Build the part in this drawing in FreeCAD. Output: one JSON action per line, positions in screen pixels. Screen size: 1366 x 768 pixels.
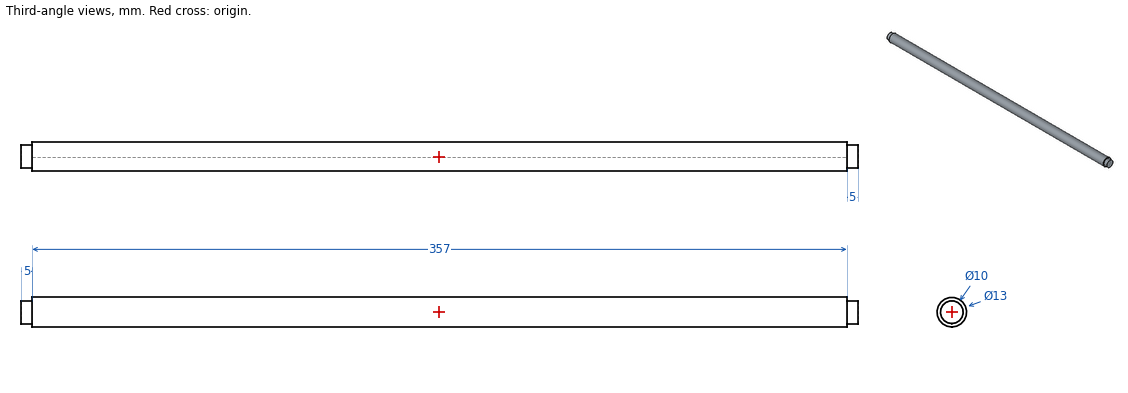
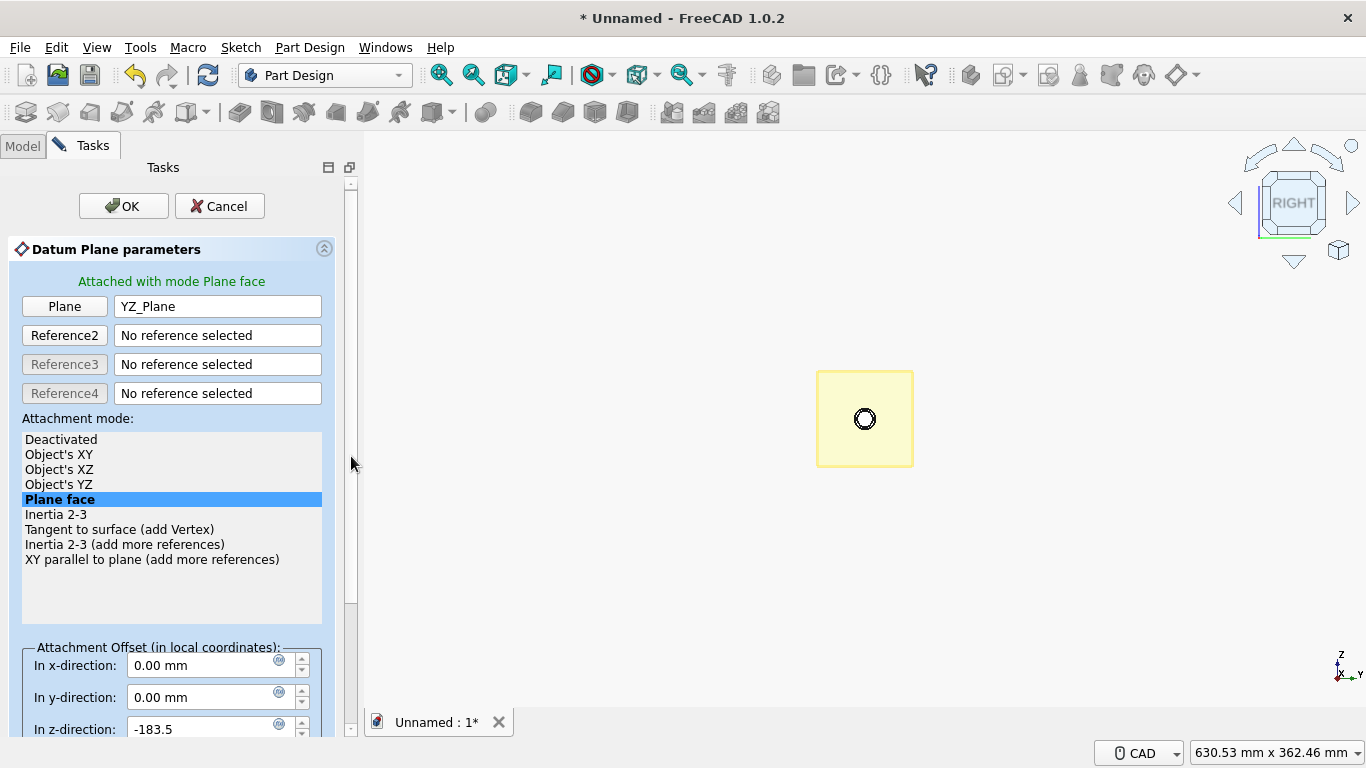
{"action": "left_click", "coordinate": [124, 206]}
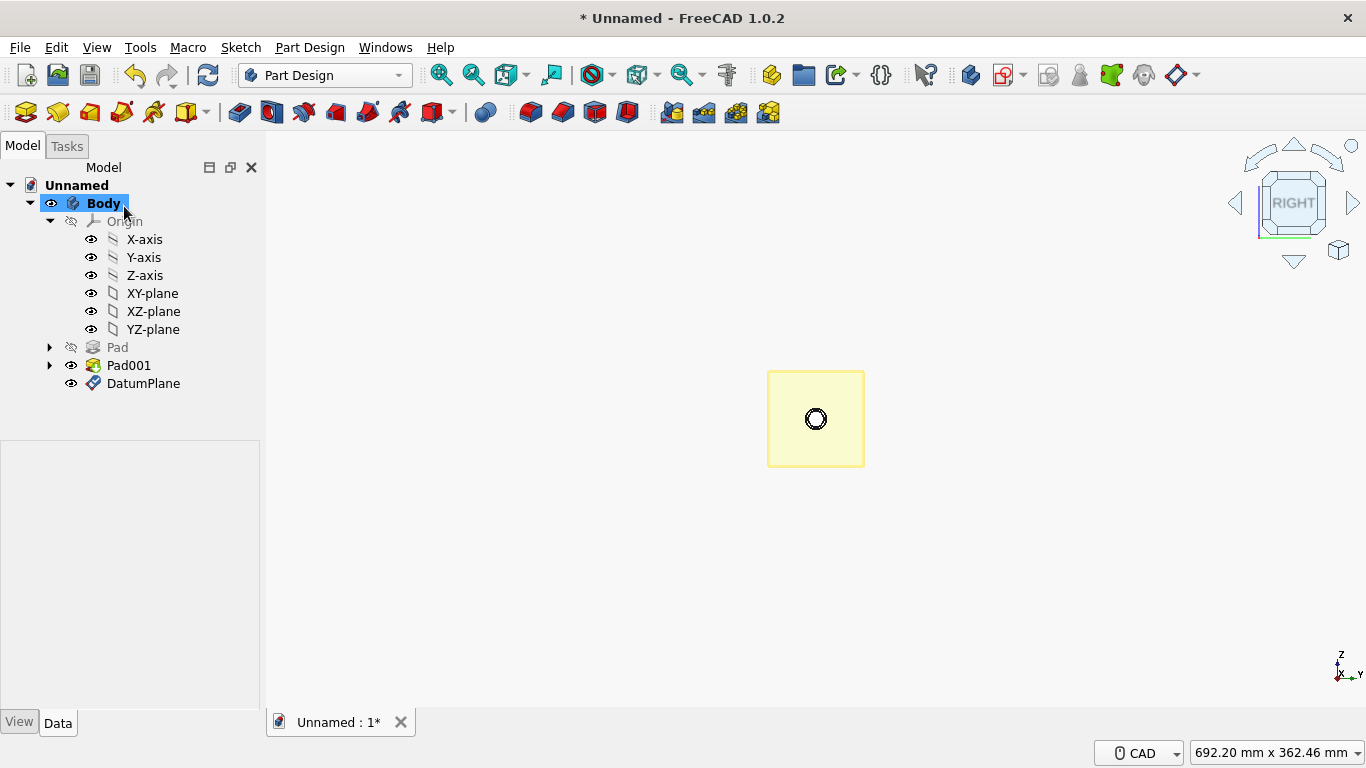
{"action": "left_click", "coordinate": [116, 383]}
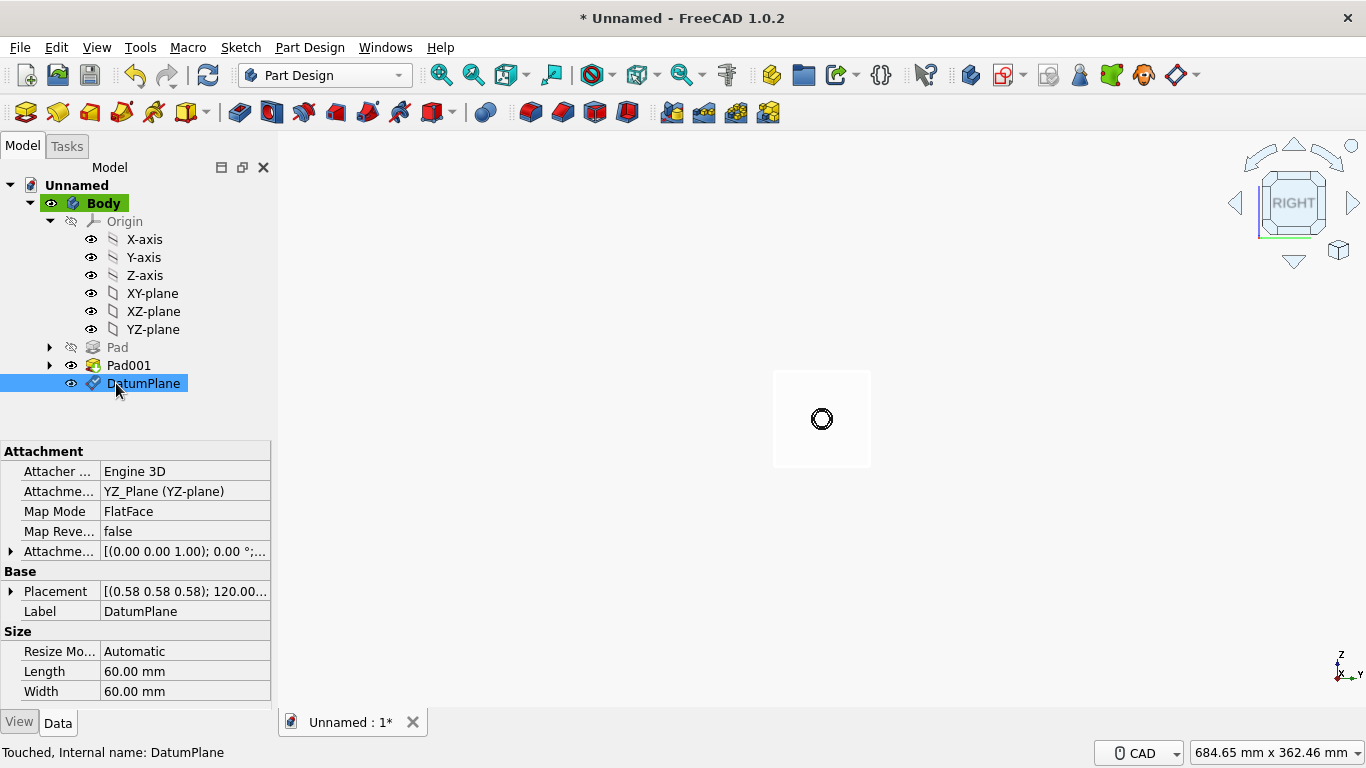
{"action": "left_click", "coordinate": [1004, 76]}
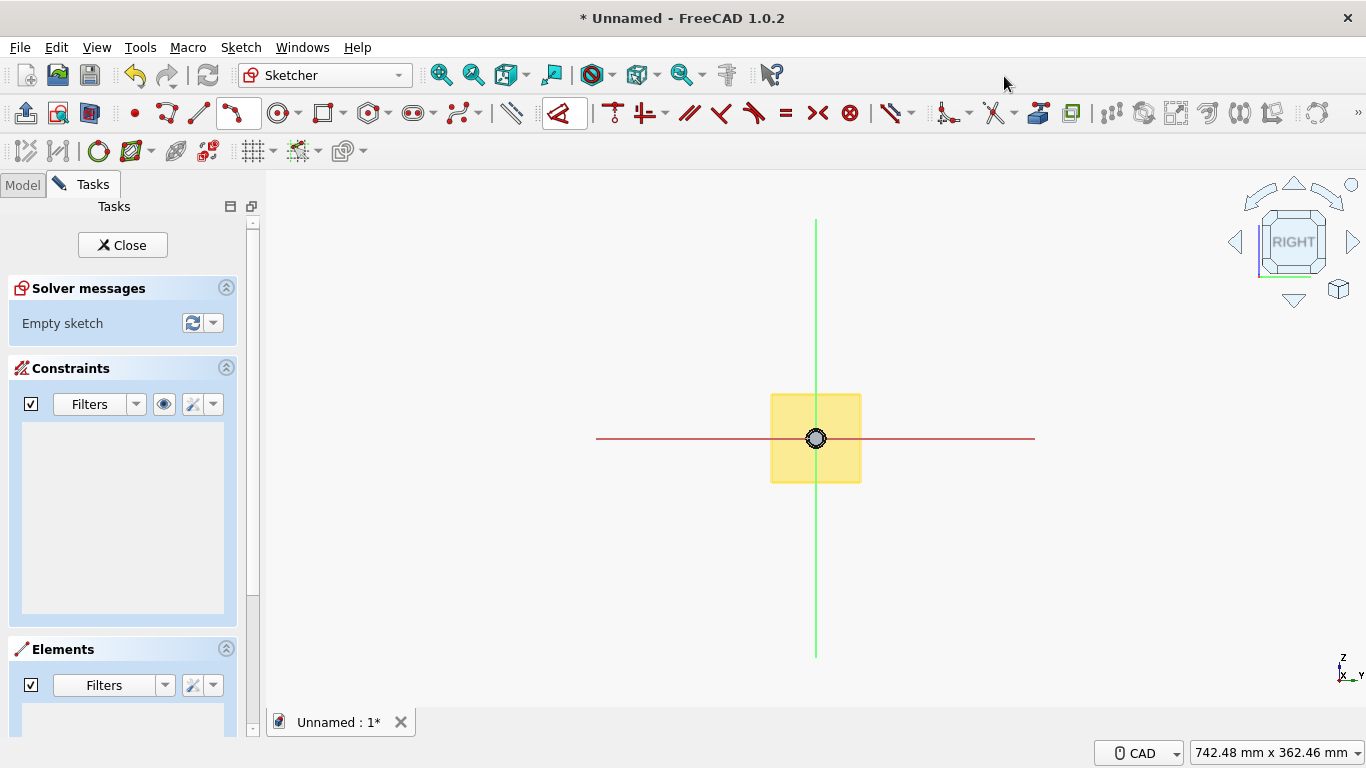
{"action": "left_click", "coordinate": [90, 114]}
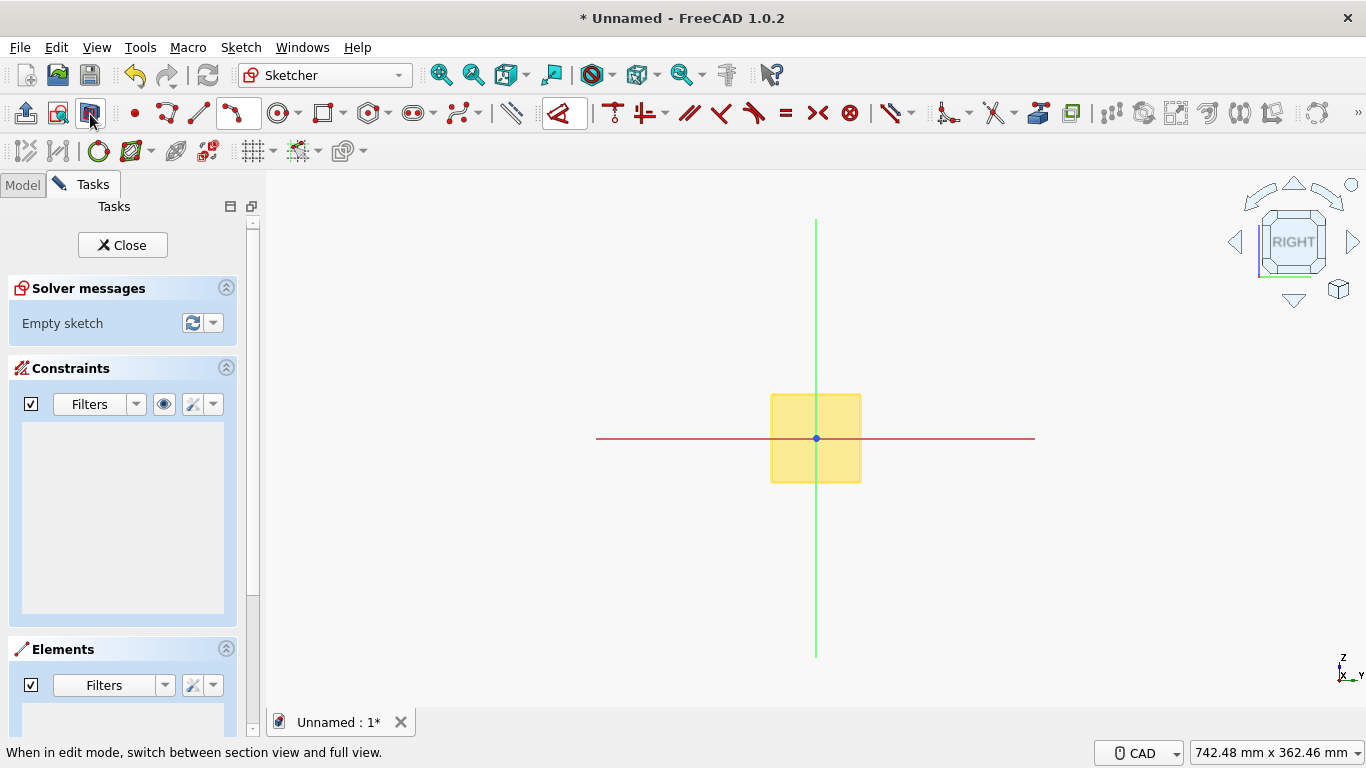
{"action": "scroll", "coordinate": [820, 438], "scroll_direction": "up", "scroll_amount": 15}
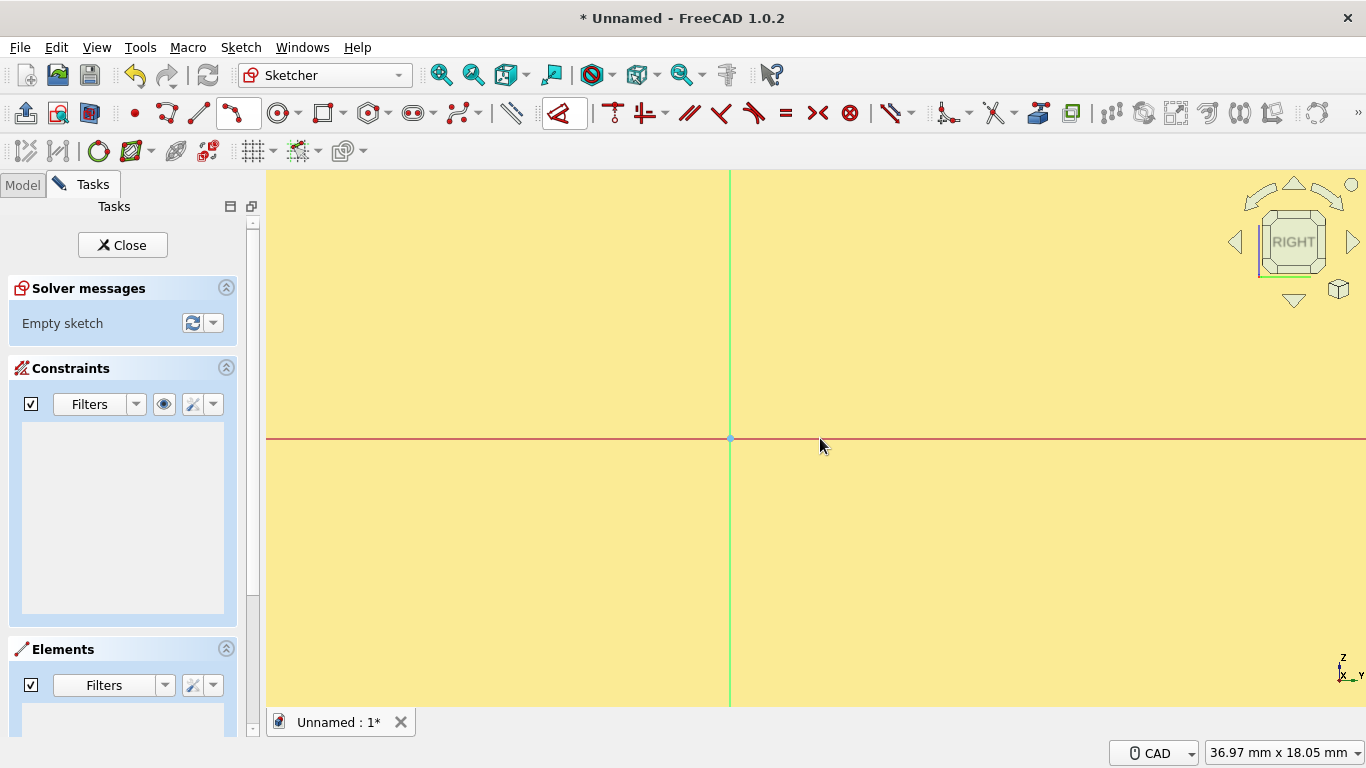
{"action": "left_click", "coordinate": [278, 114]}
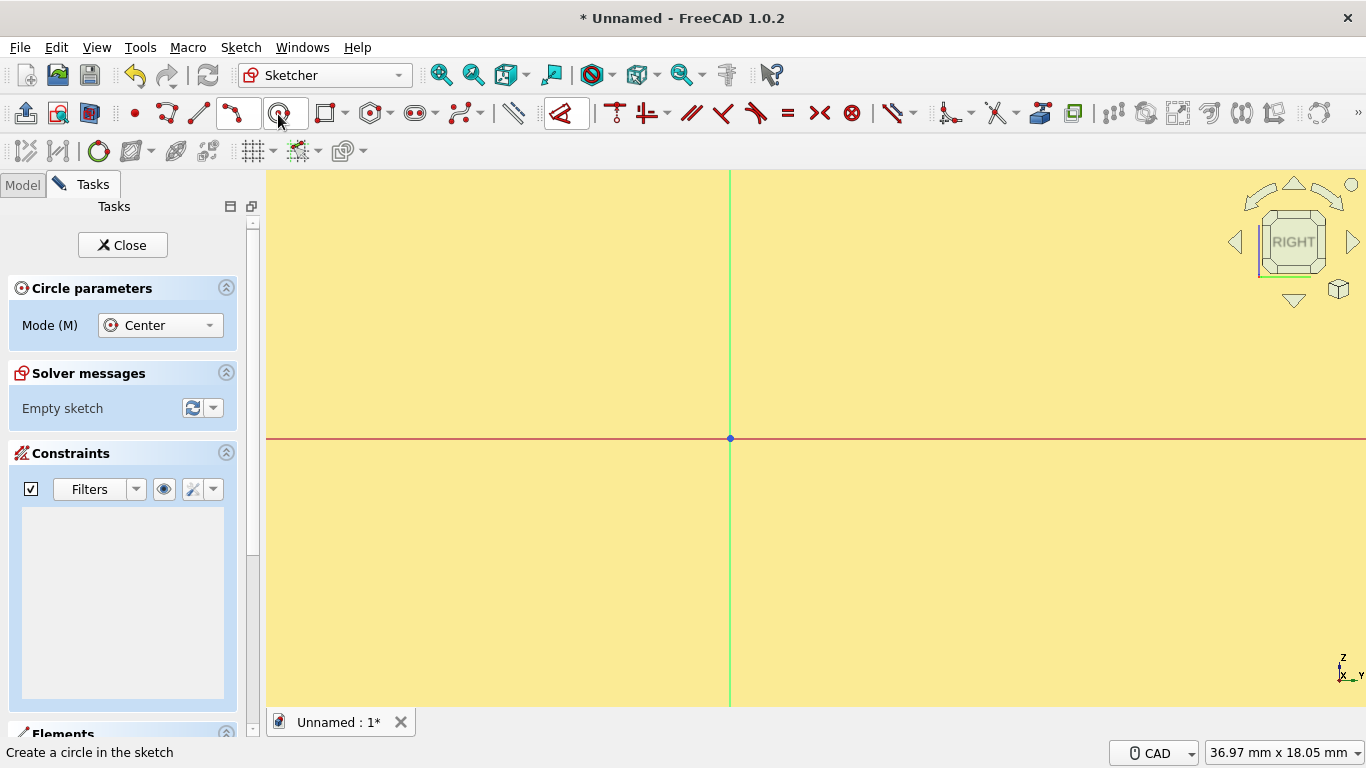
{"action": "left_click", "coordinate": [730, 438]}
{"action": "left_click", "coordinate": [835, 333]}
{"action": "key", "text": "Escape"}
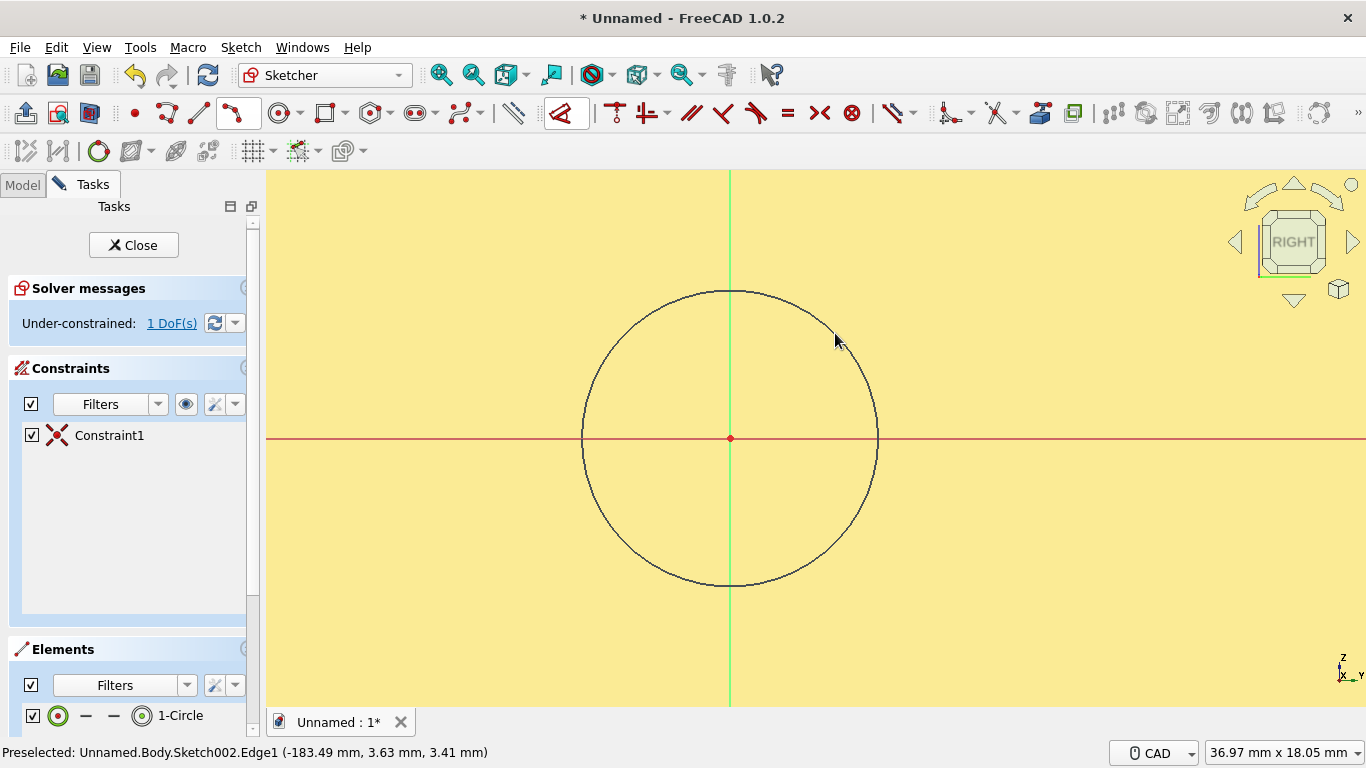
{"action": "left_click", "coordinate": [834, 333]}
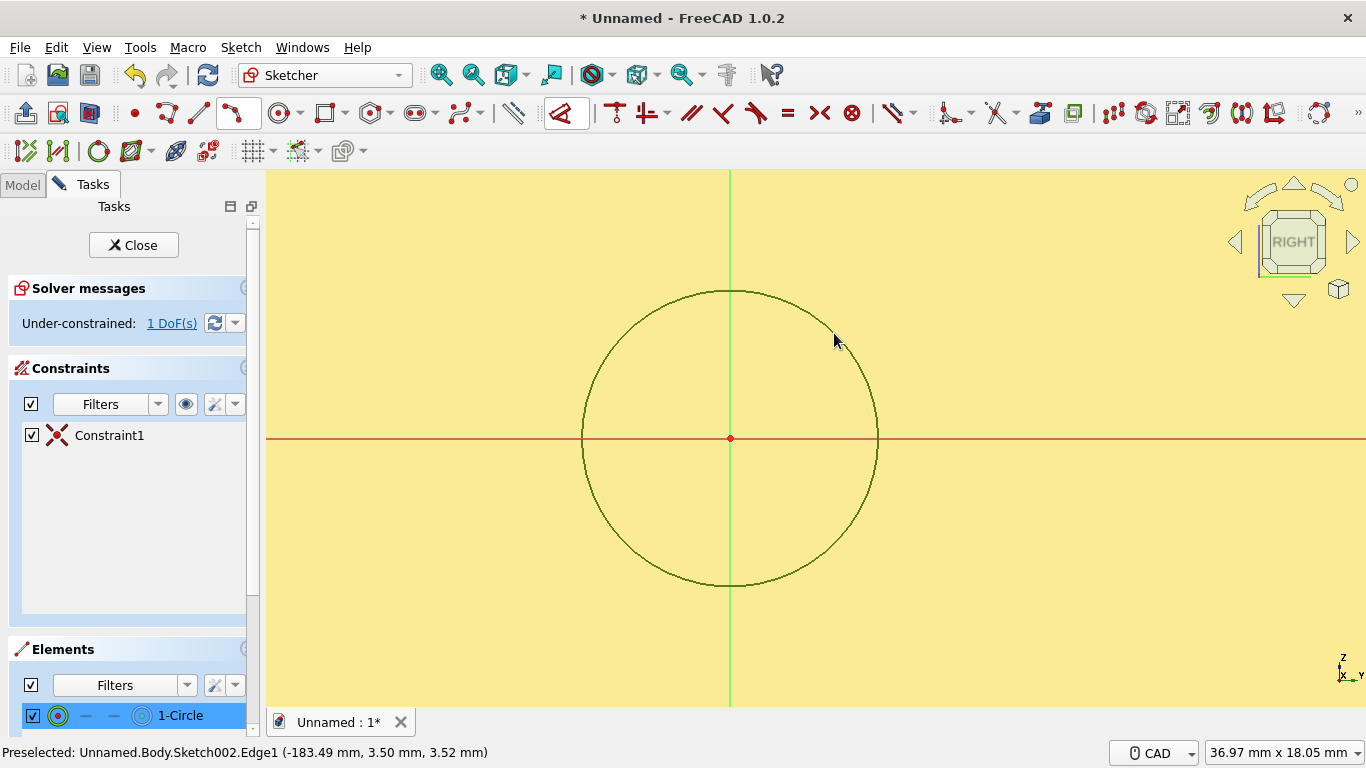
{"action": "left_click", "coordinate": [584, 114]}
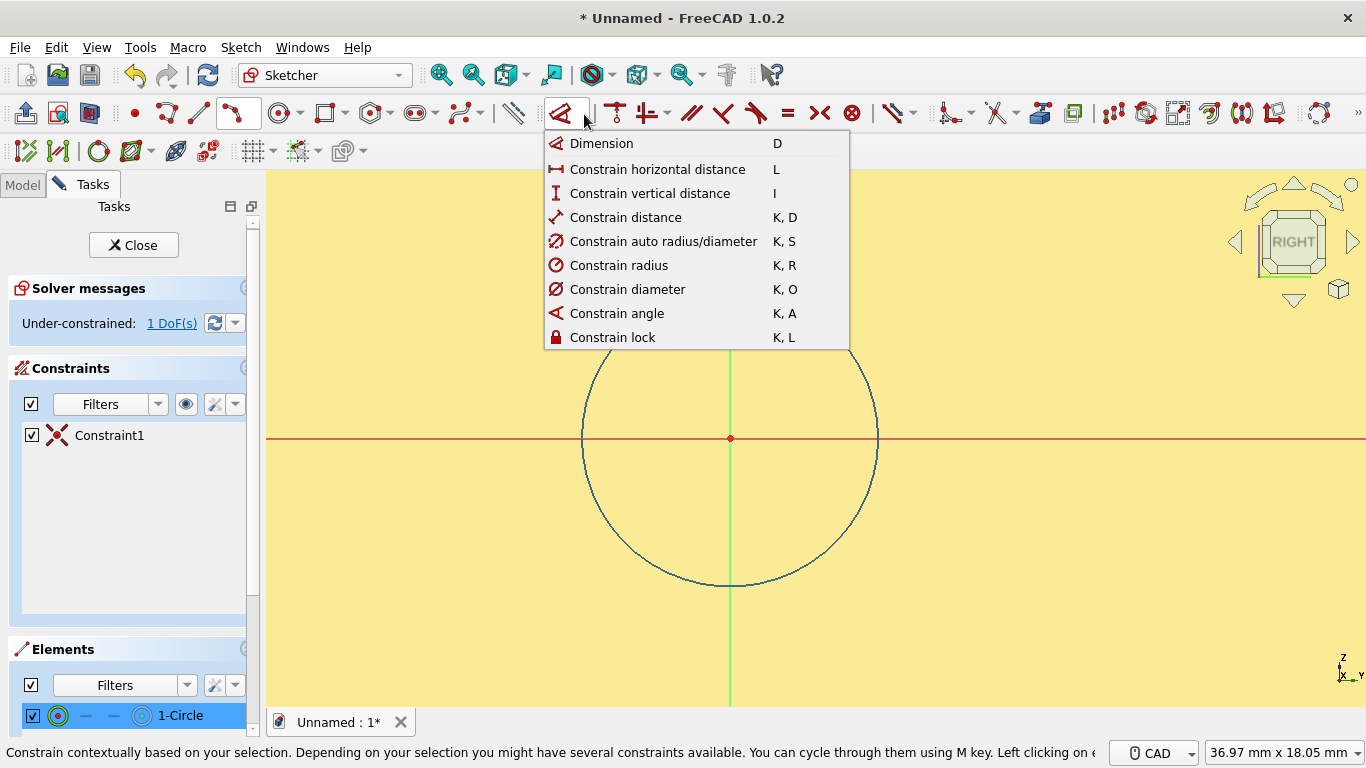
{"action": "left_click", "coordinate": [697, 289]}